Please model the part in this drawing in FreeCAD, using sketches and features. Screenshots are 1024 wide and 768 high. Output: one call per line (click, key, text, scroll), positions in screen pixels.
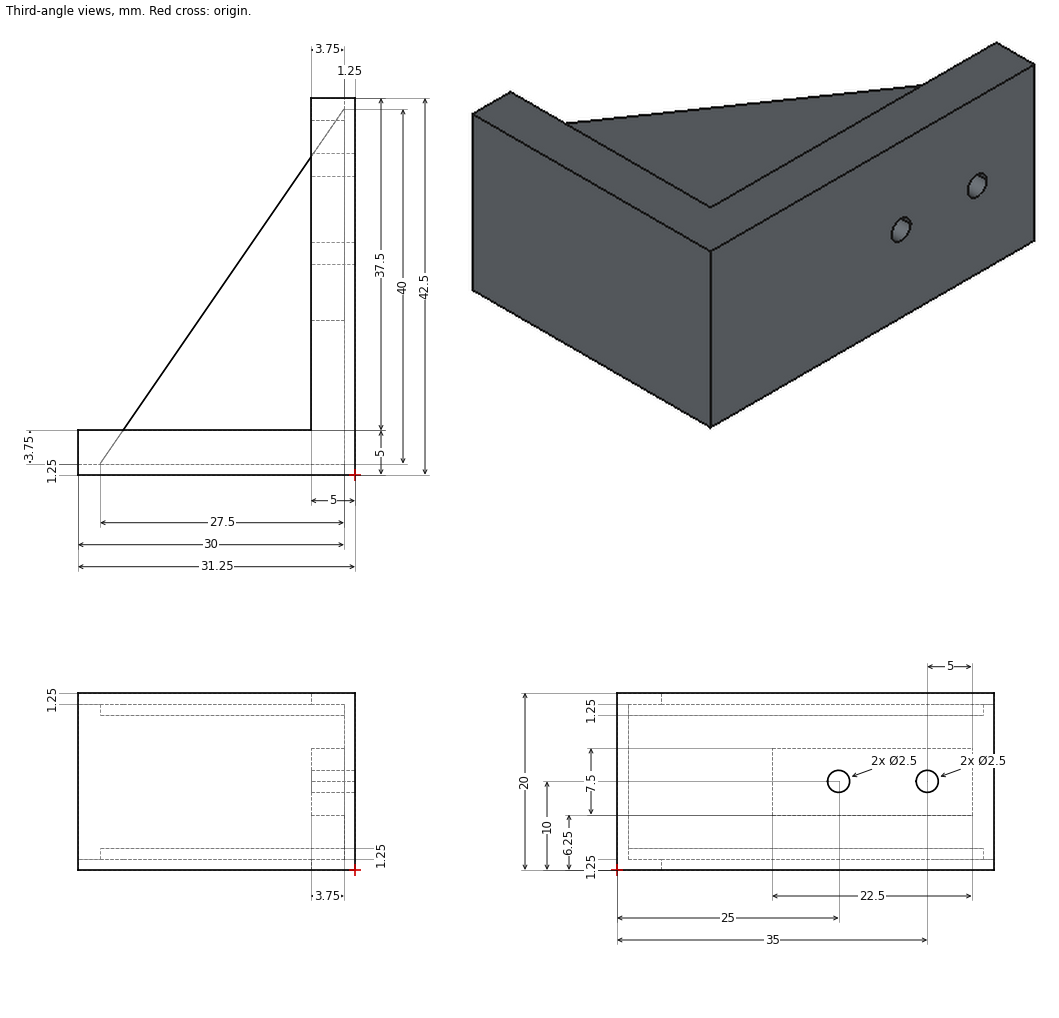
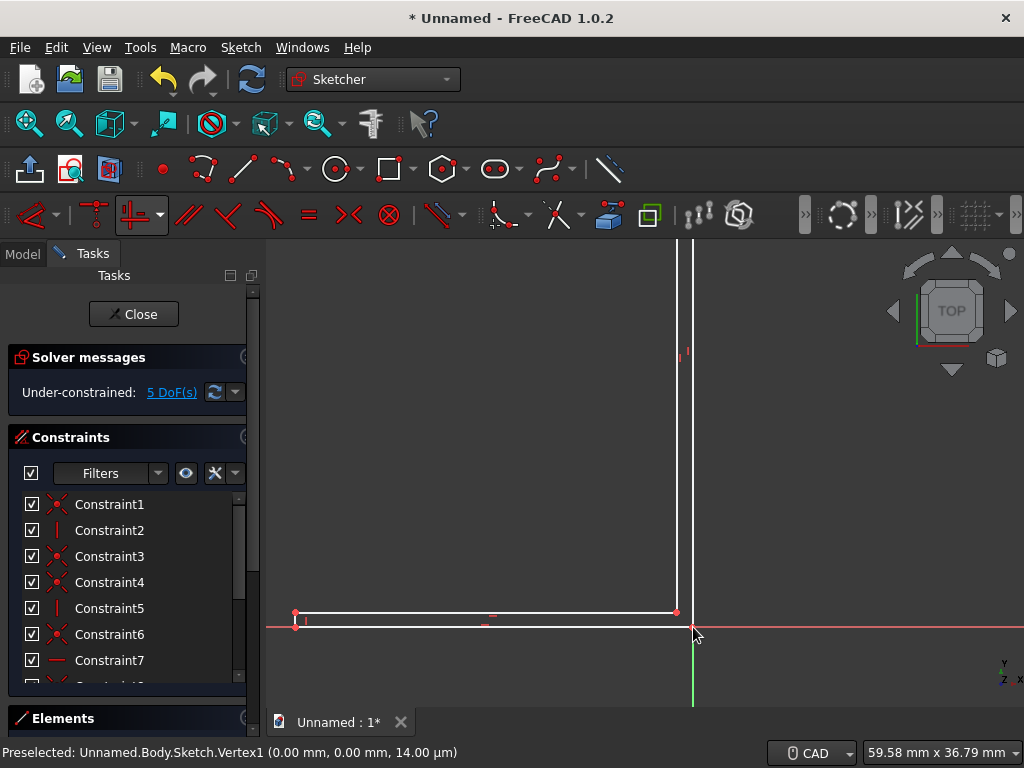
scroll(677, 614, down, 3)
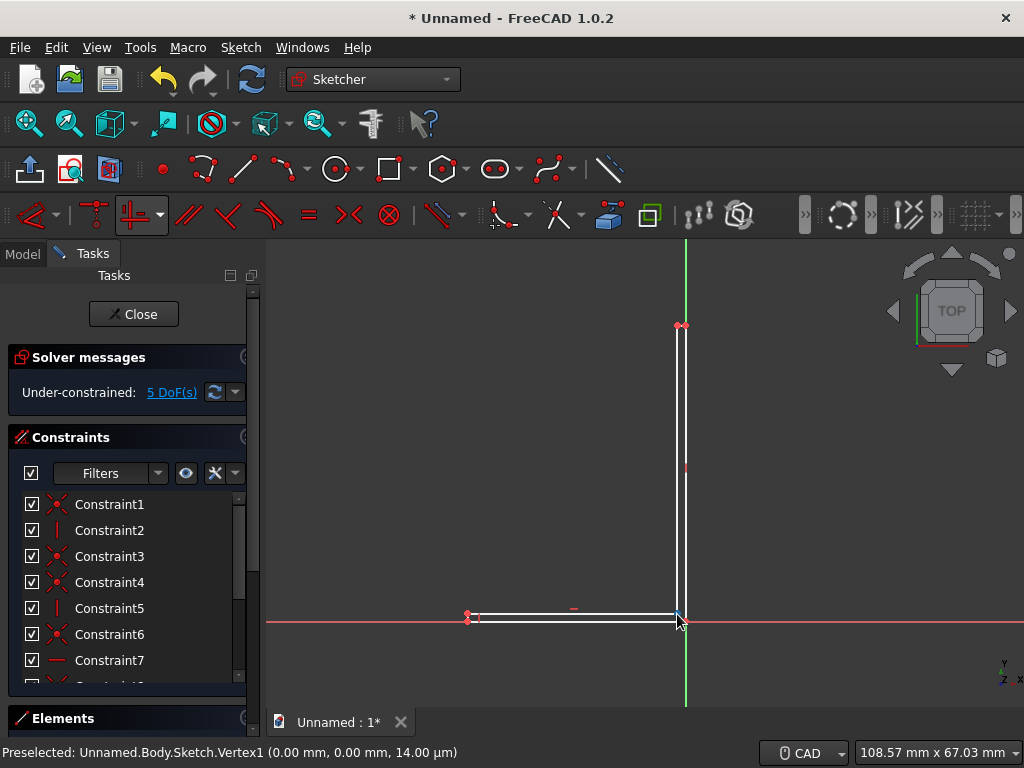
scroll(681, 326, up, 6)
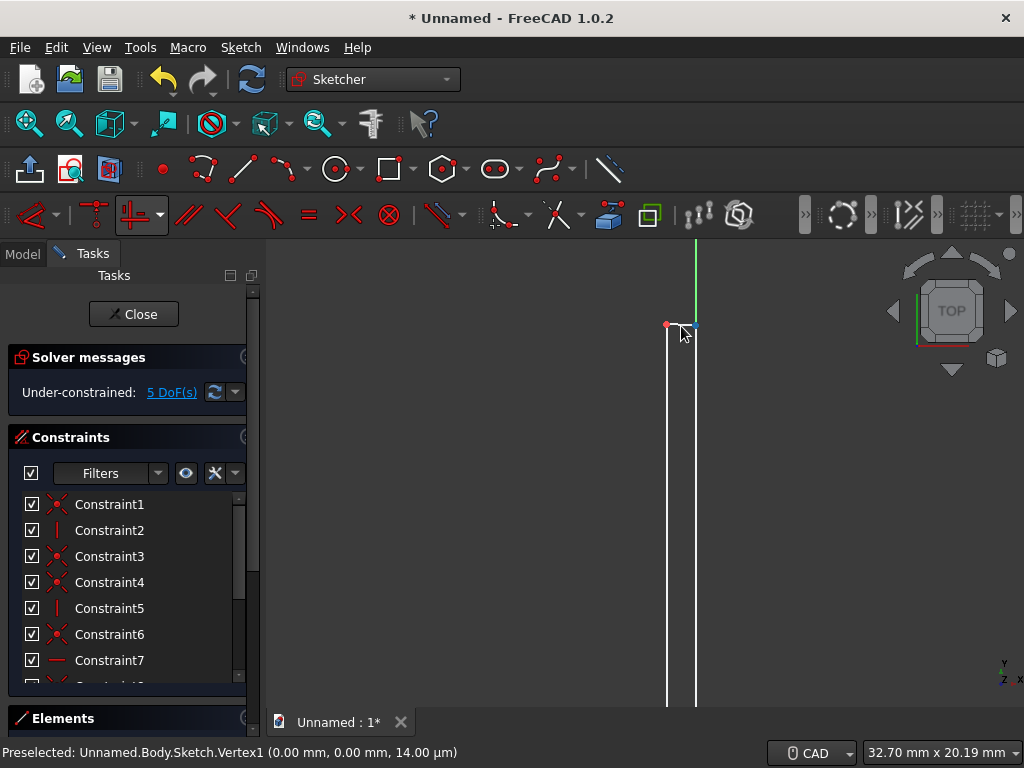
click(681, 325)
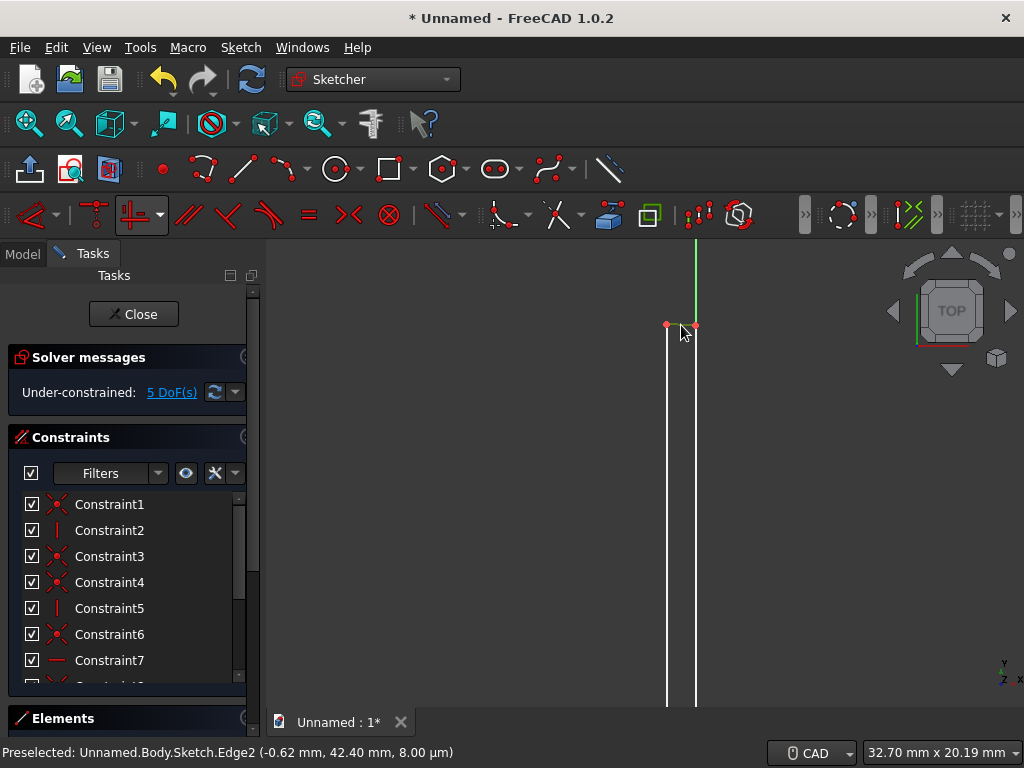
key(h)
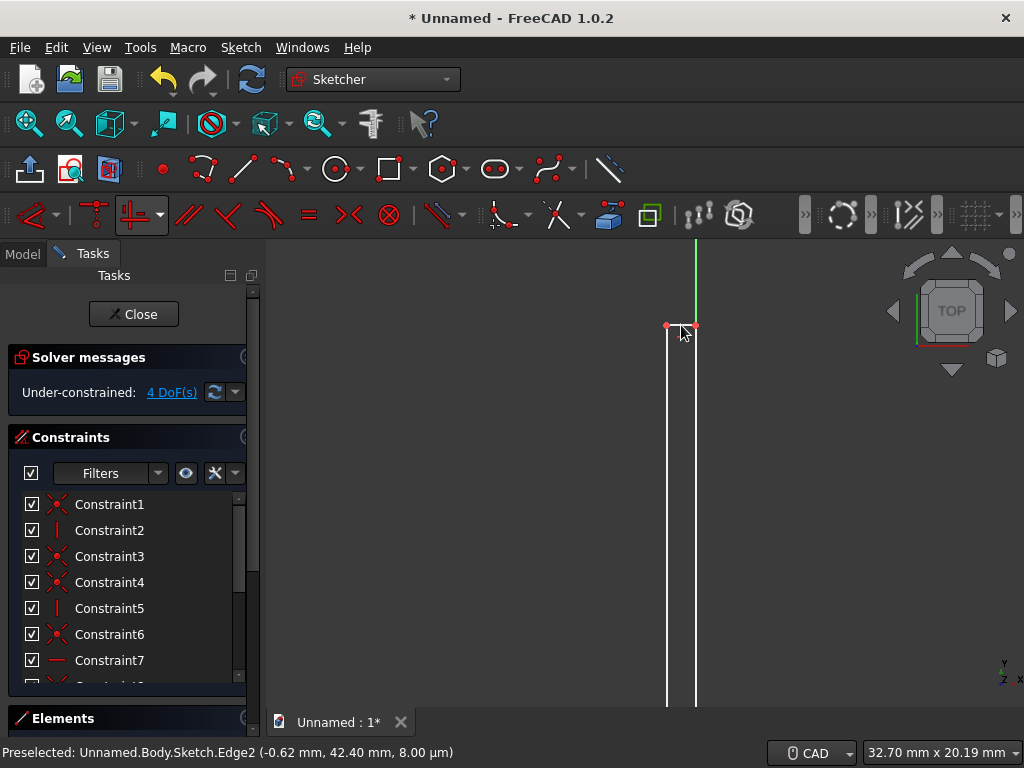
click(32, 216)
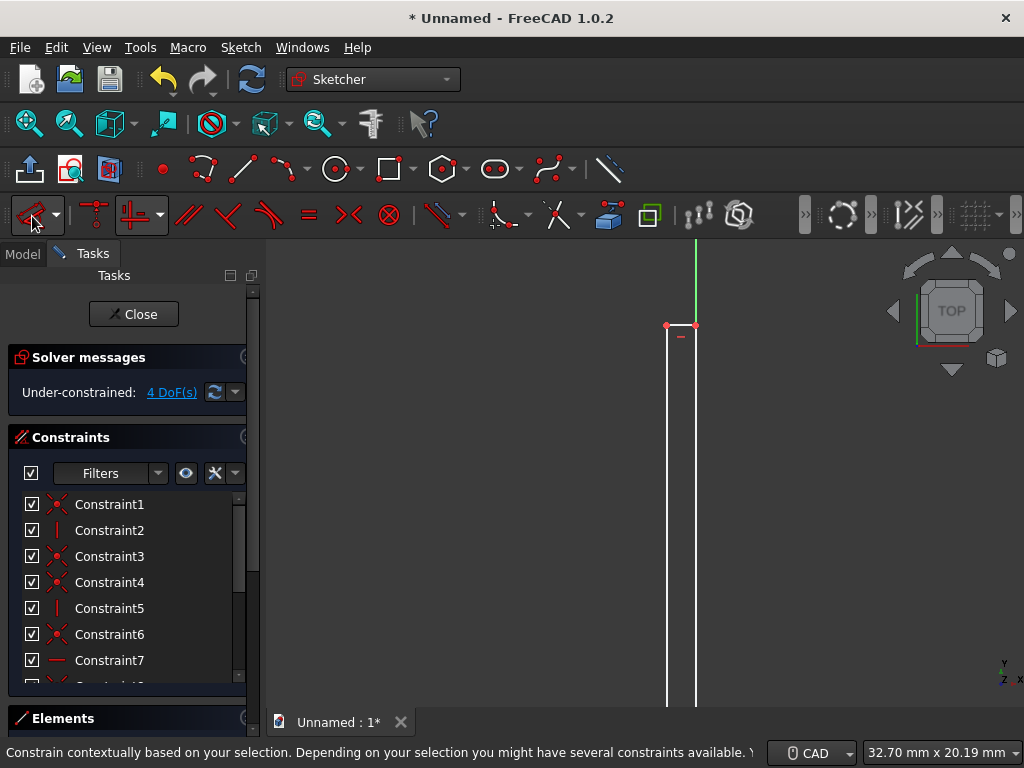
scroll(681, 326, down, 6)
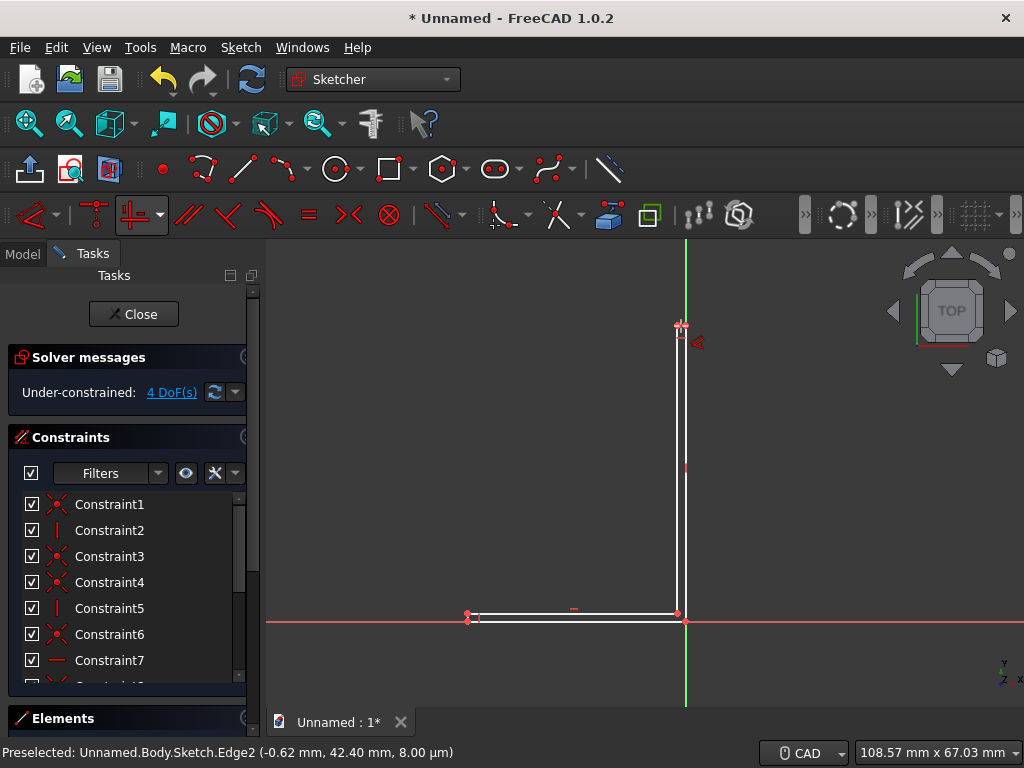
scroll(614, 614, up, 3)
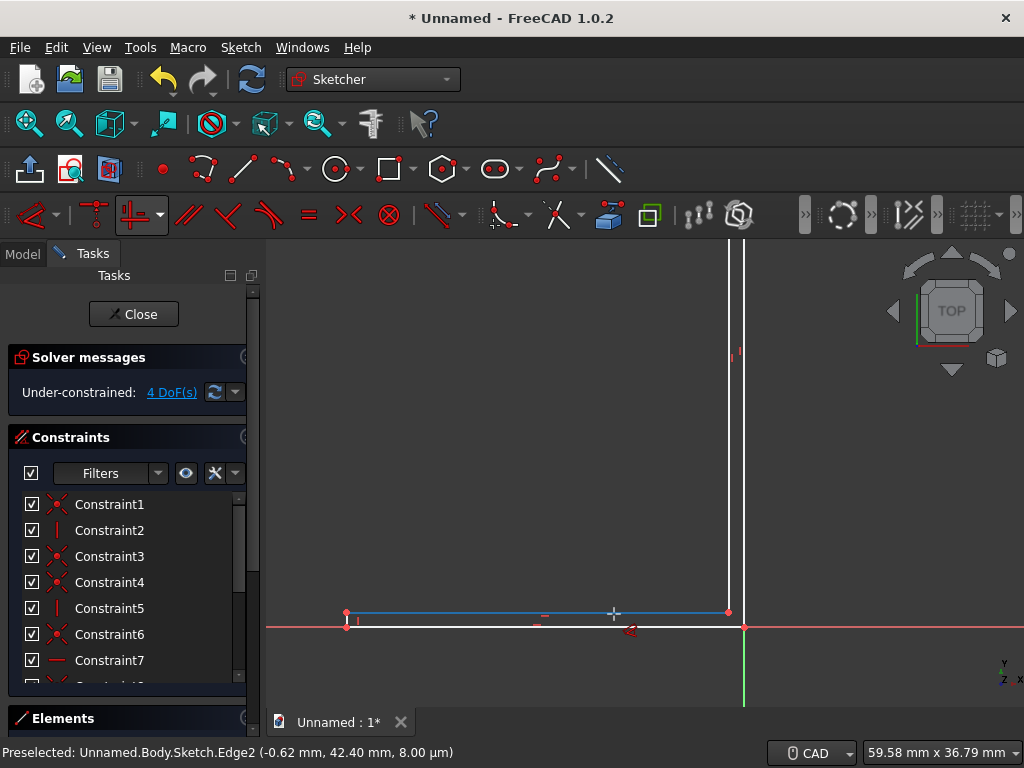
click(614, 613)
click(538, 647)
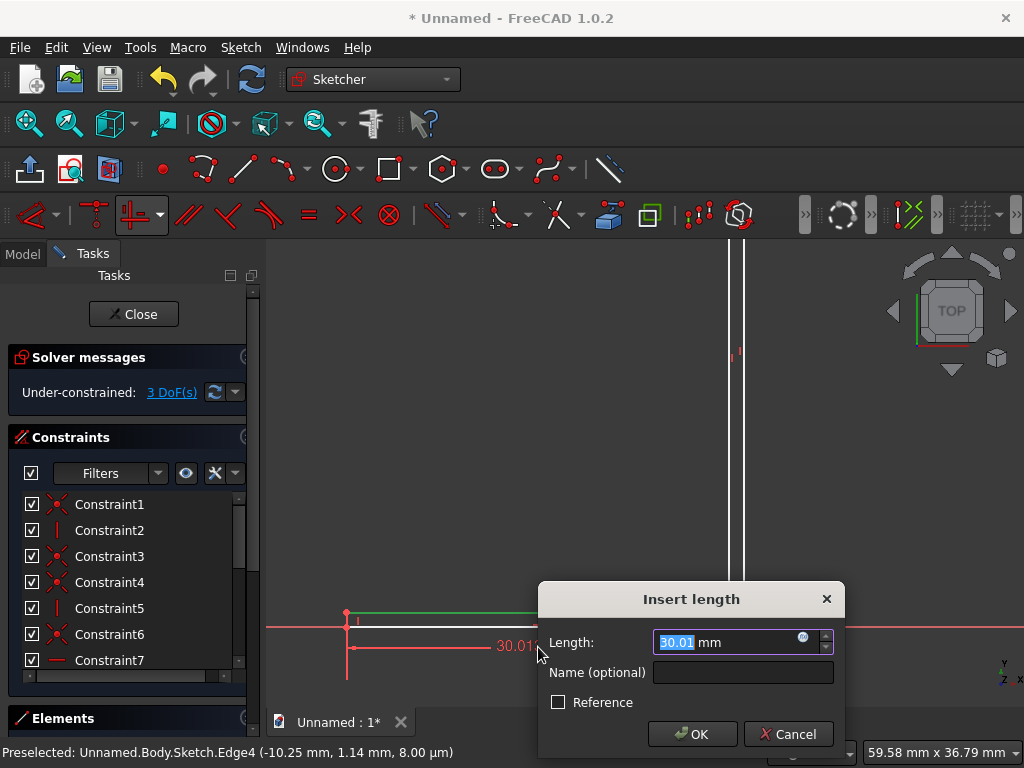
text(30)
key(Return)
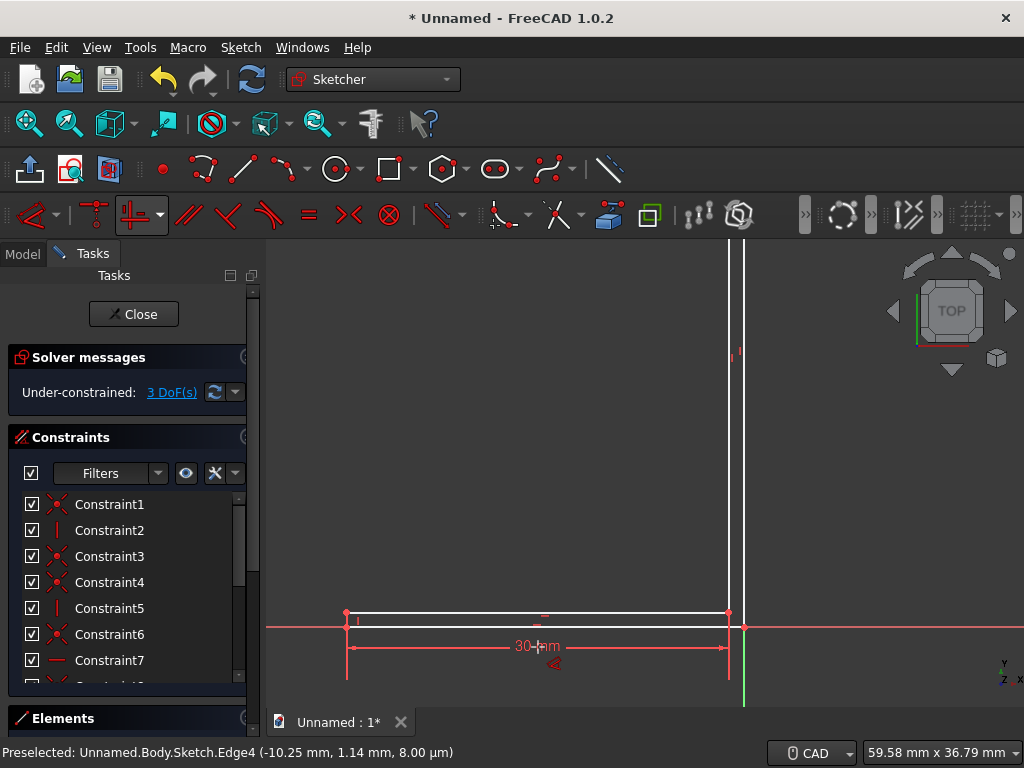
click(744, 466)
click(778, 447)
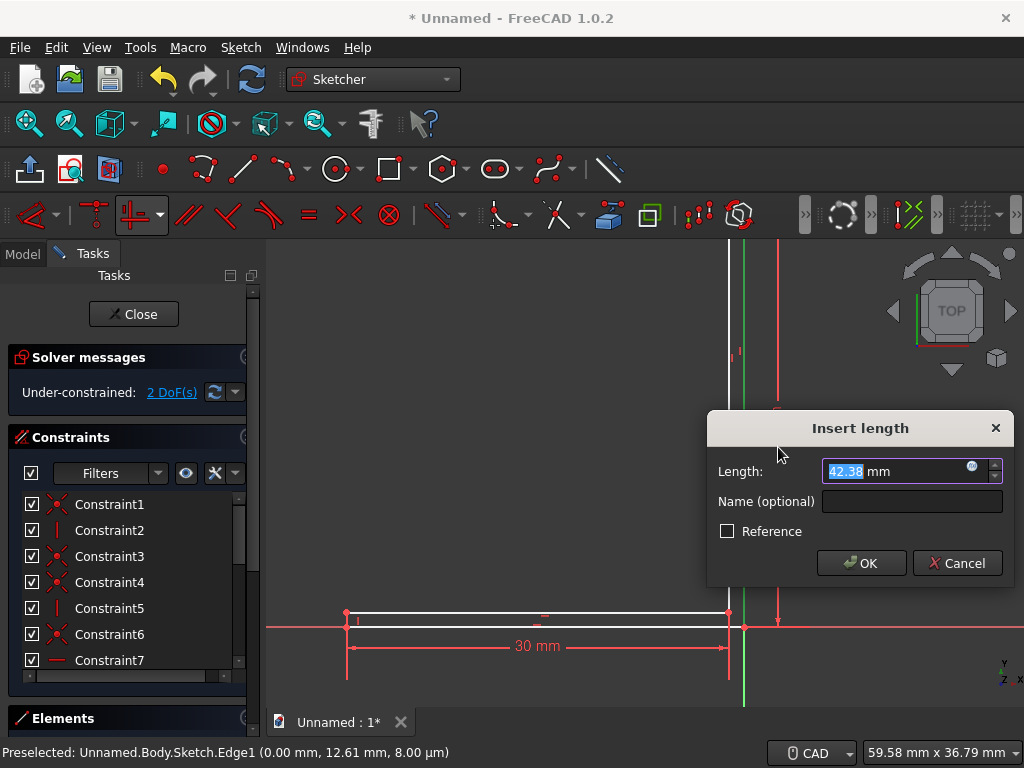
text(42.5)
key(Return)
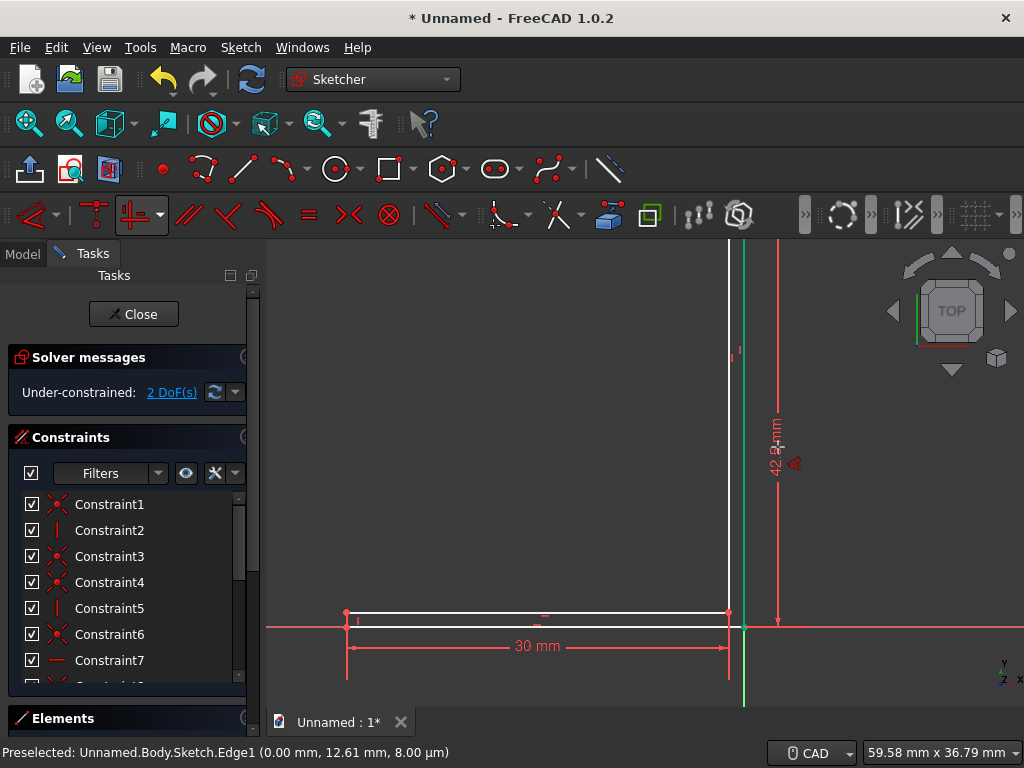
scroll(614, 614, down, 3)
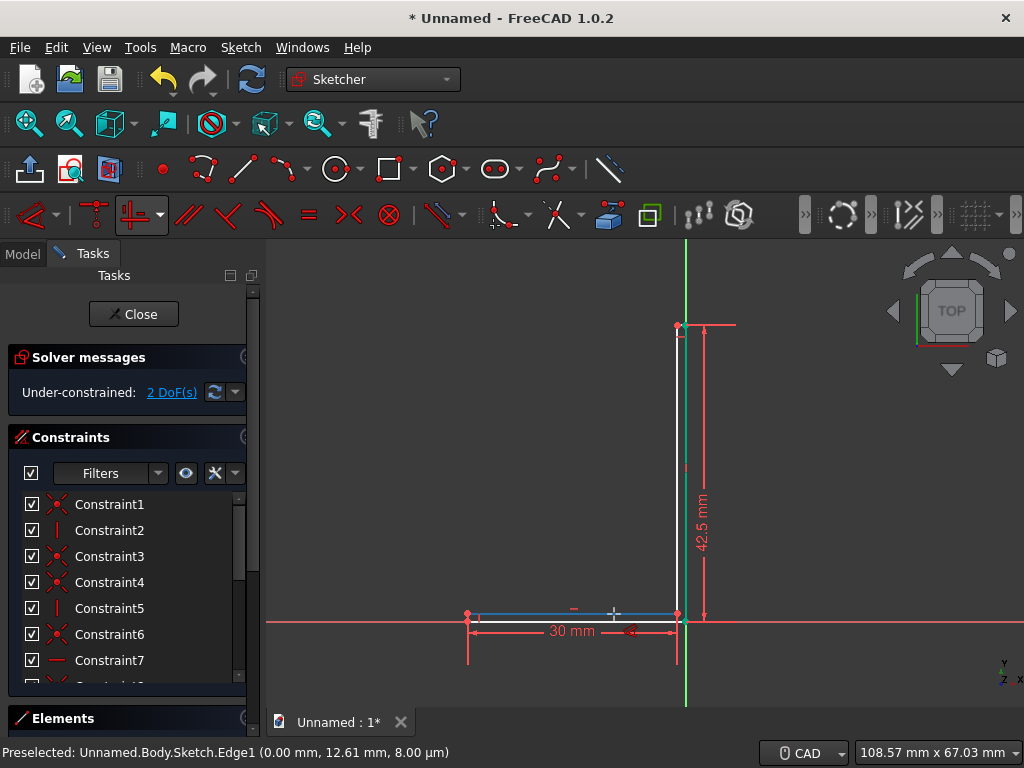
scroll(681, 325, up, 8)